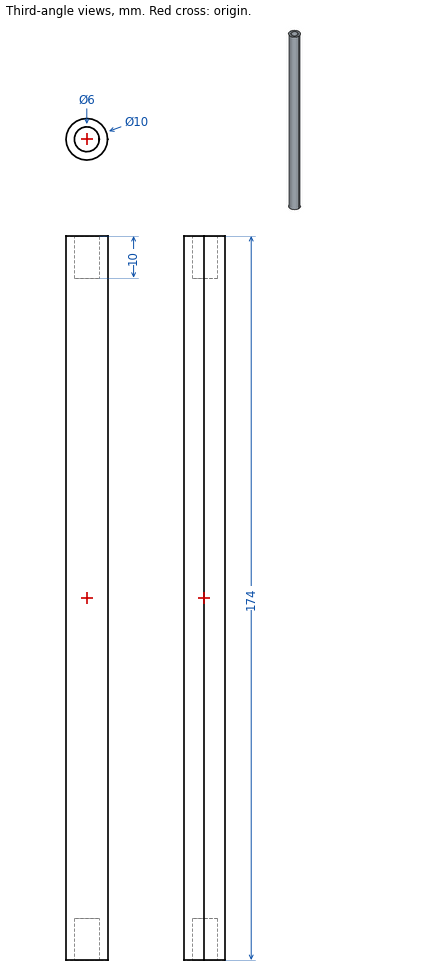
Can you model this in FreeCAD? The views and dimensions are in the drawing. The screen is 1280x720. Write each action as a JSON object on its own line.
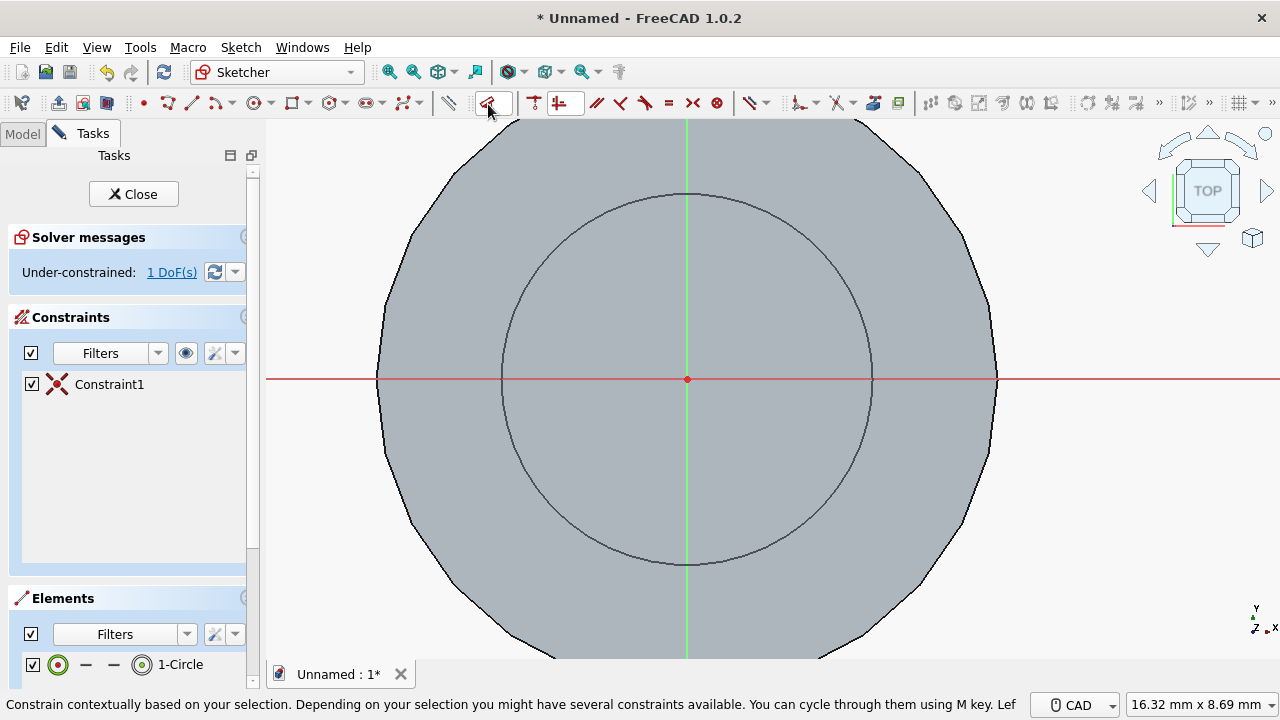
{"action": "left_click", "coordinate": [818, 248]}
{"action": "left_click", "coordinate": [841, 225]}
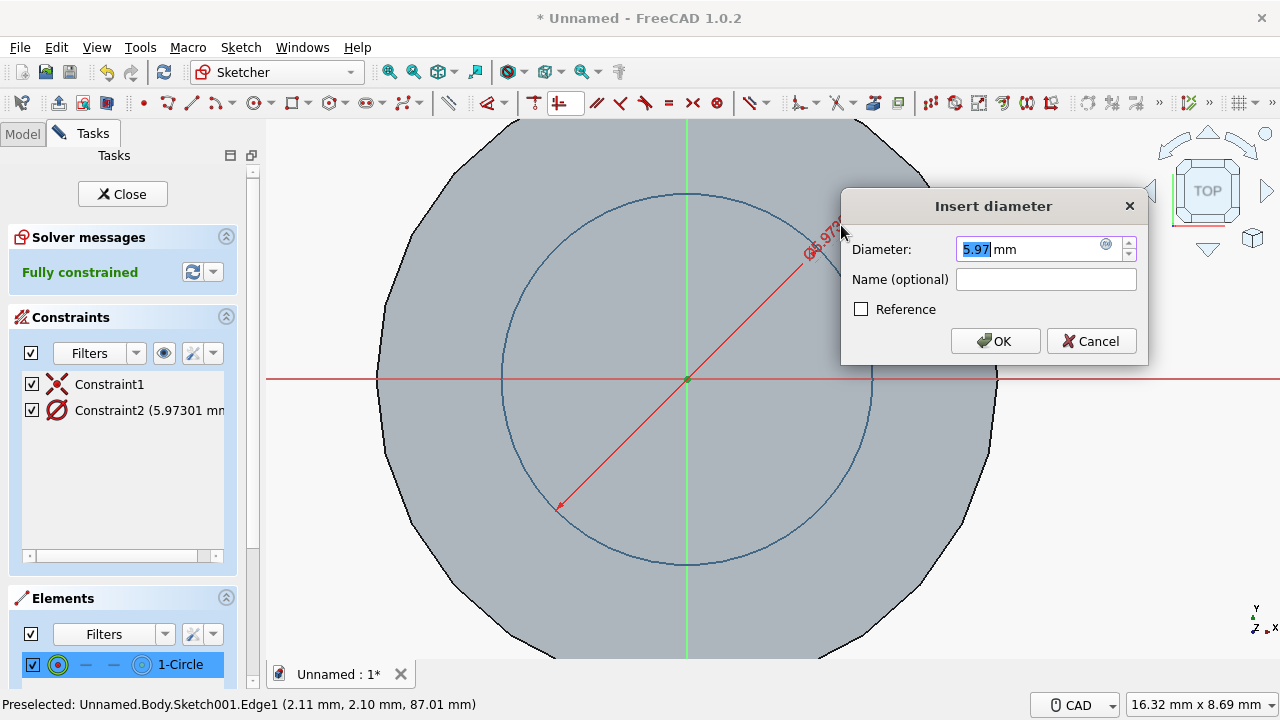
{"action": "type", "text": "6"}
{"action": "key", "text": "Return"}
{"action": "key", "text": "Escape"}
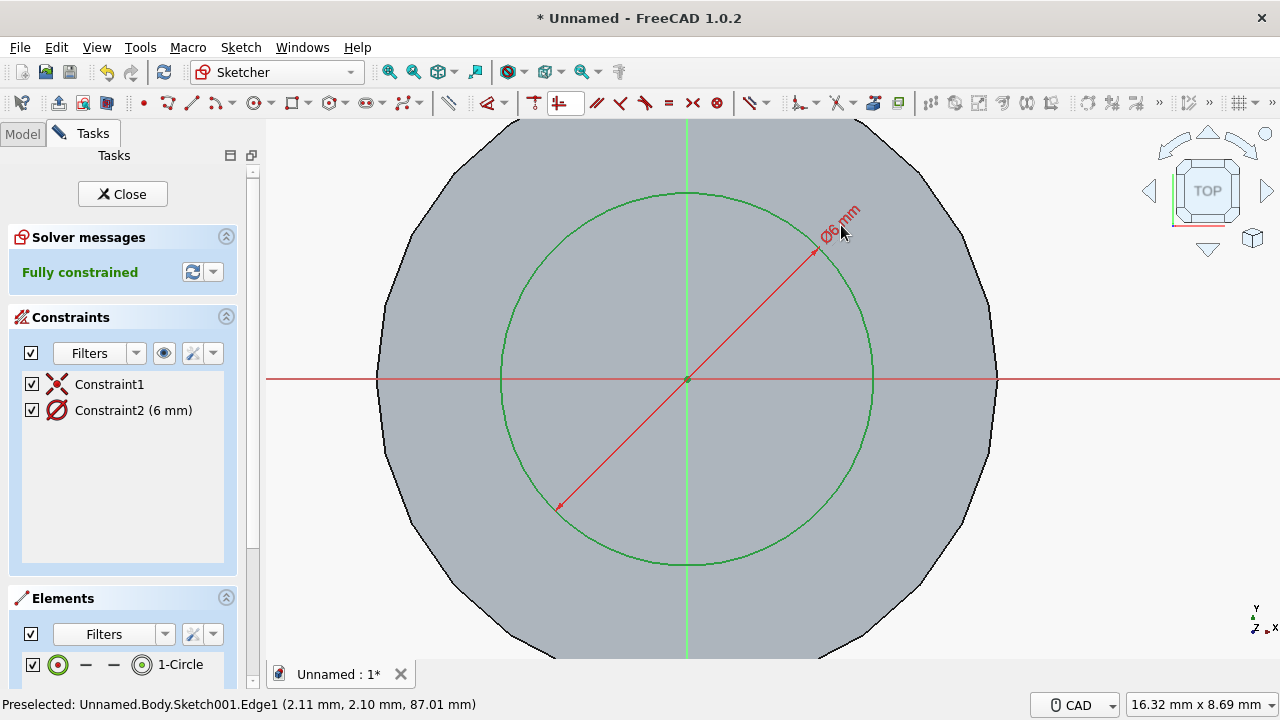
{"action": "left_click", "coordinate": [123, 194]}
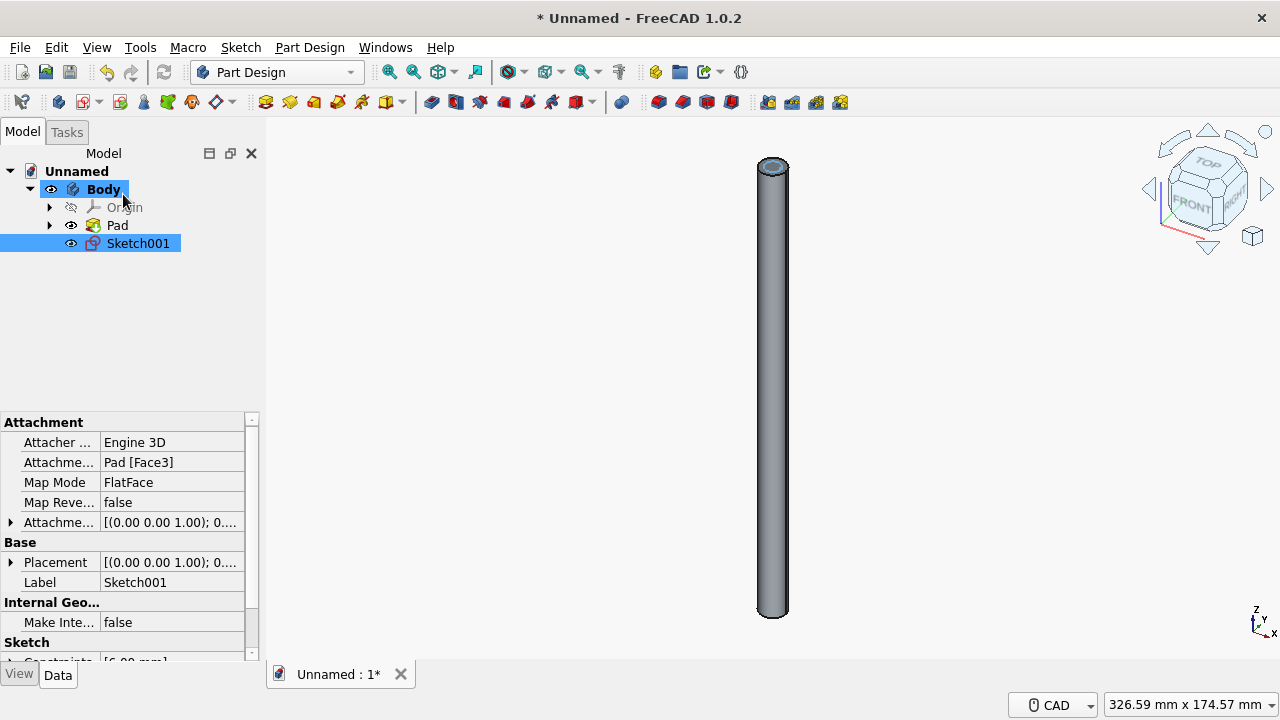
{"action": "left_click", "coordinate": [432, 102]}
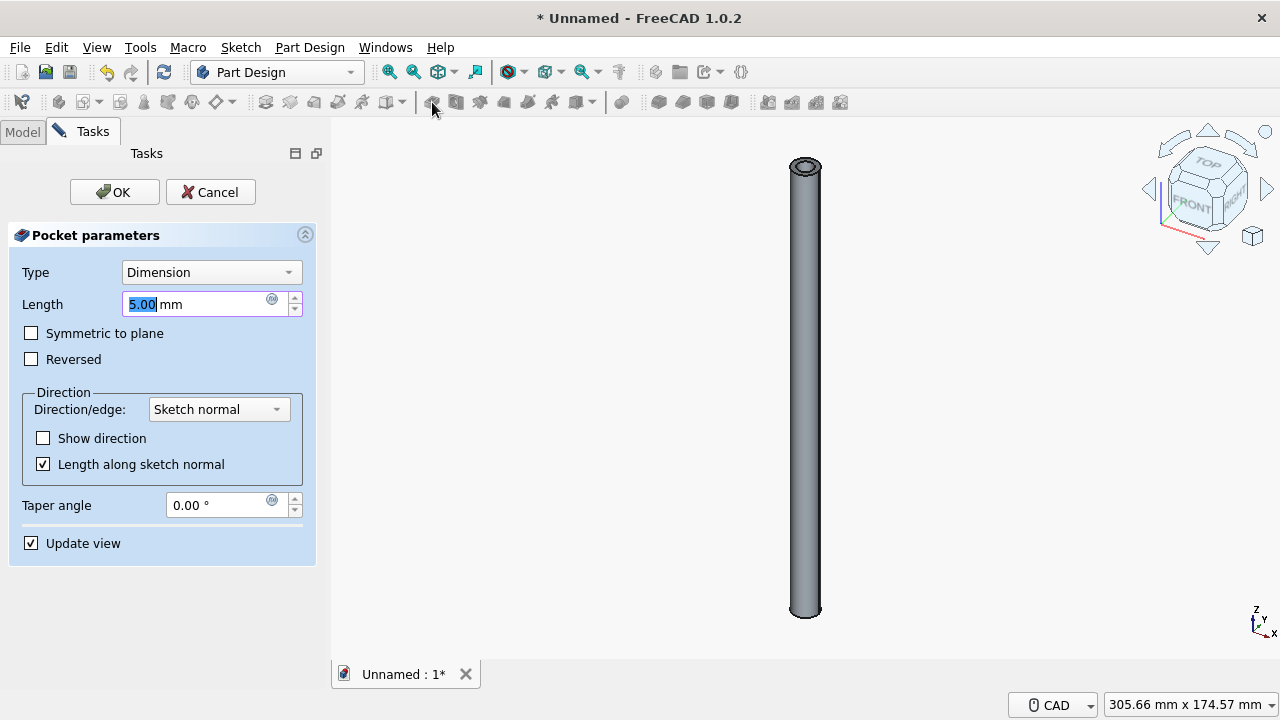
{"action": "type", "text": "10"}
{"action": "key", "text": "Tab"}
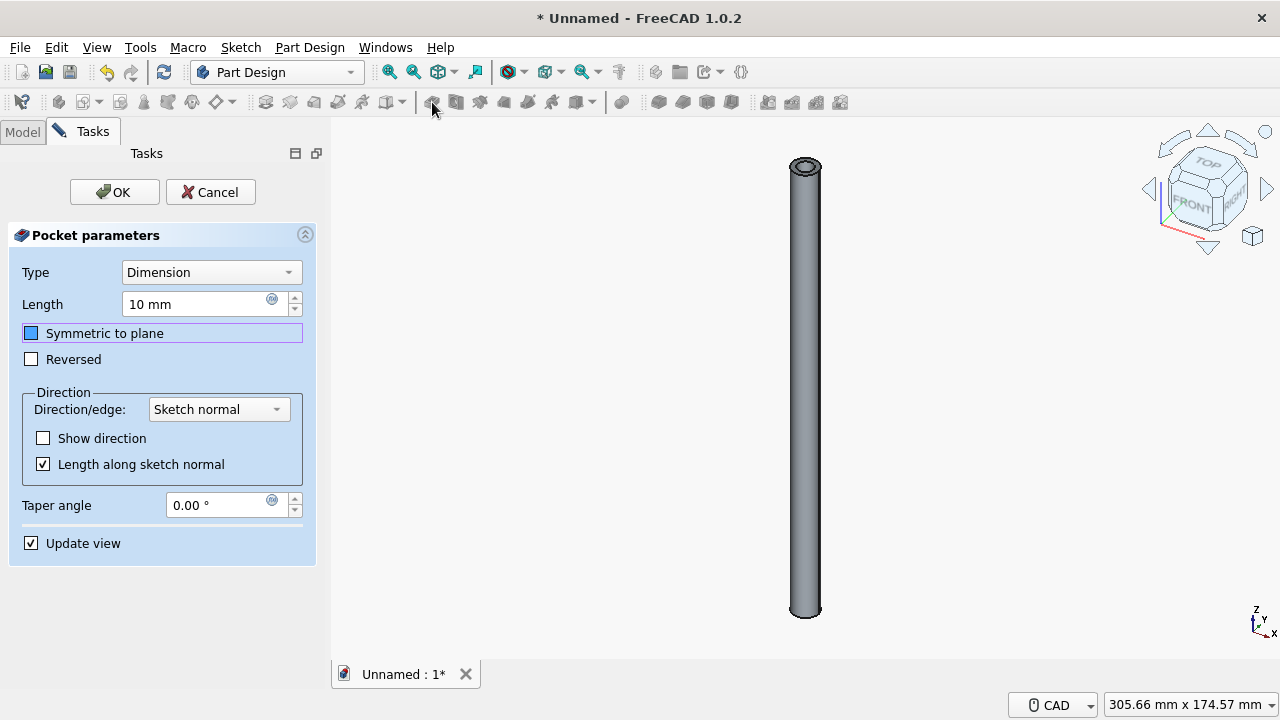
{"action": "left_click", "coordinate": [115, 192]}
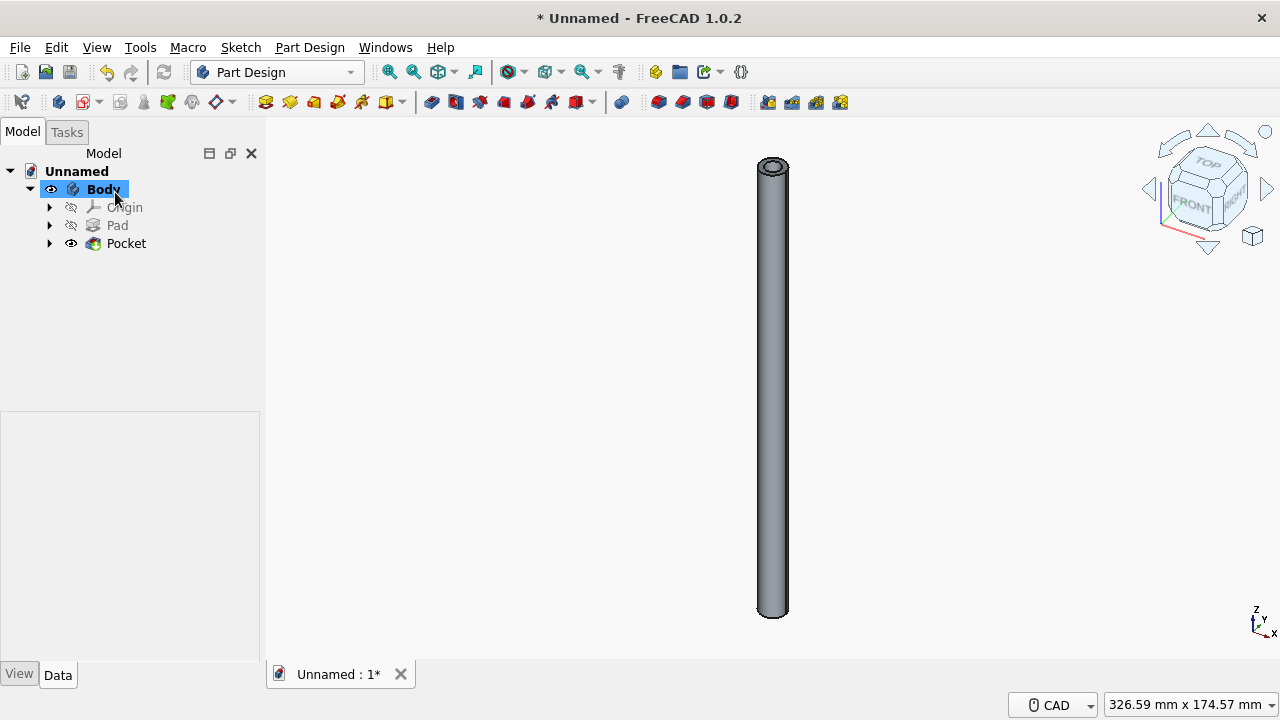
{"action": "left_click", "coordinate": [116, 243]}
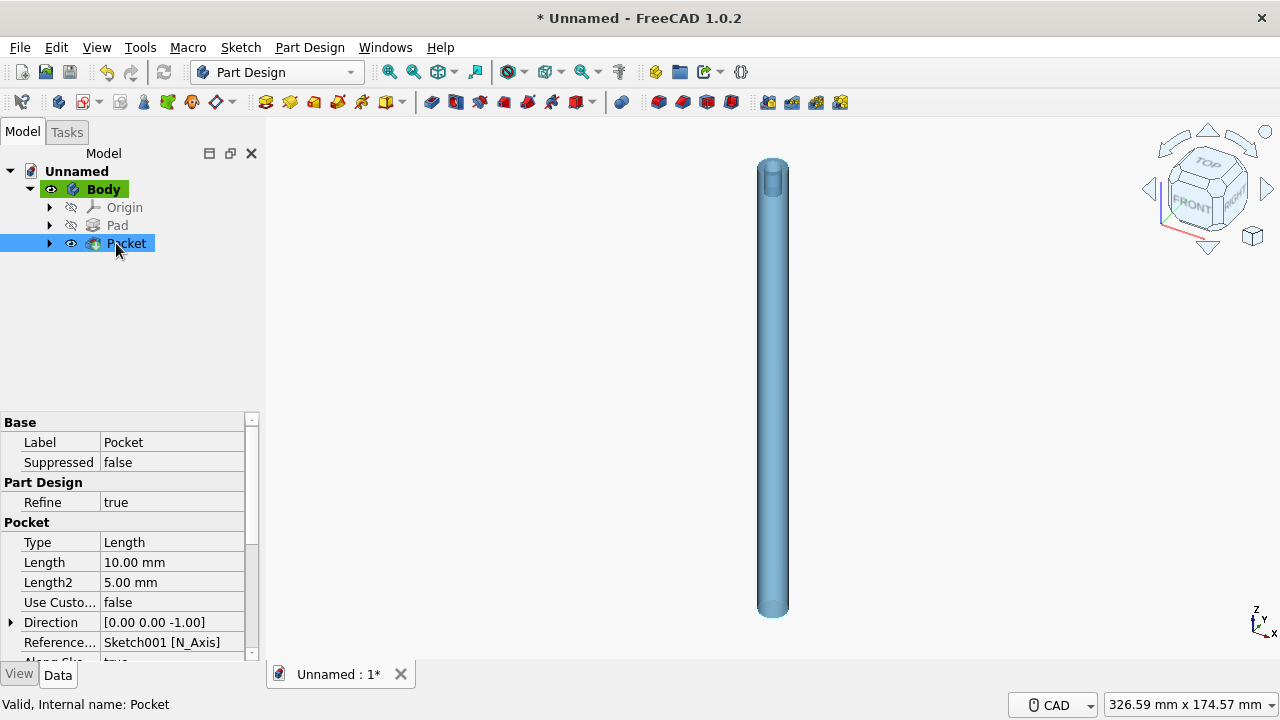
{"action": "left_click", "coordinate": [768, 102]}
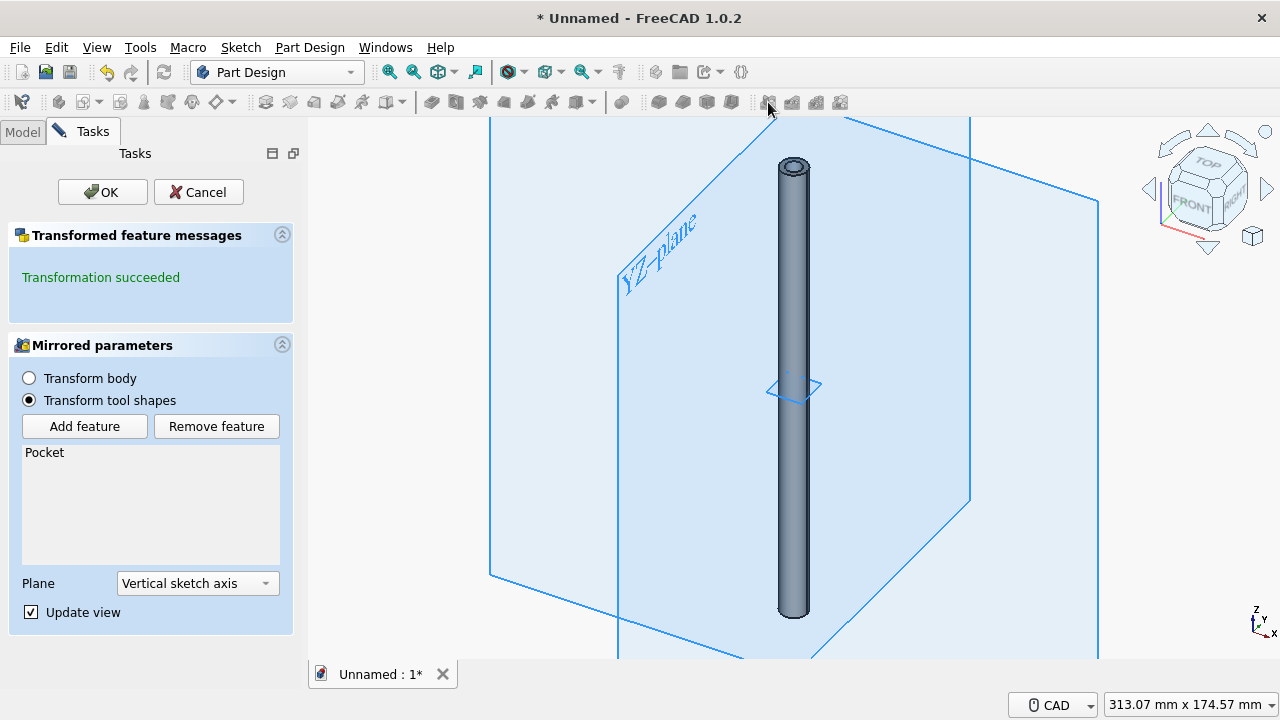
{"action": "left_click", "coordinate": [198, 584]}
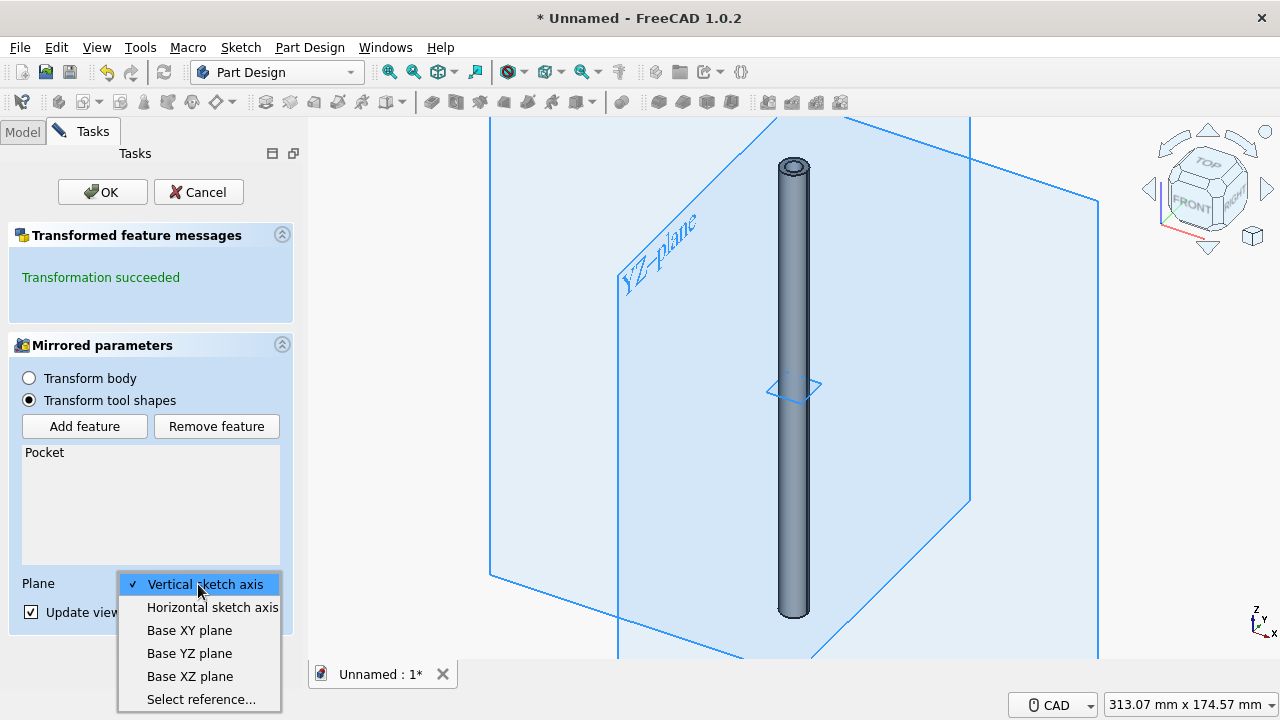
{"action": "left_click", "coordinate": [198, 630]}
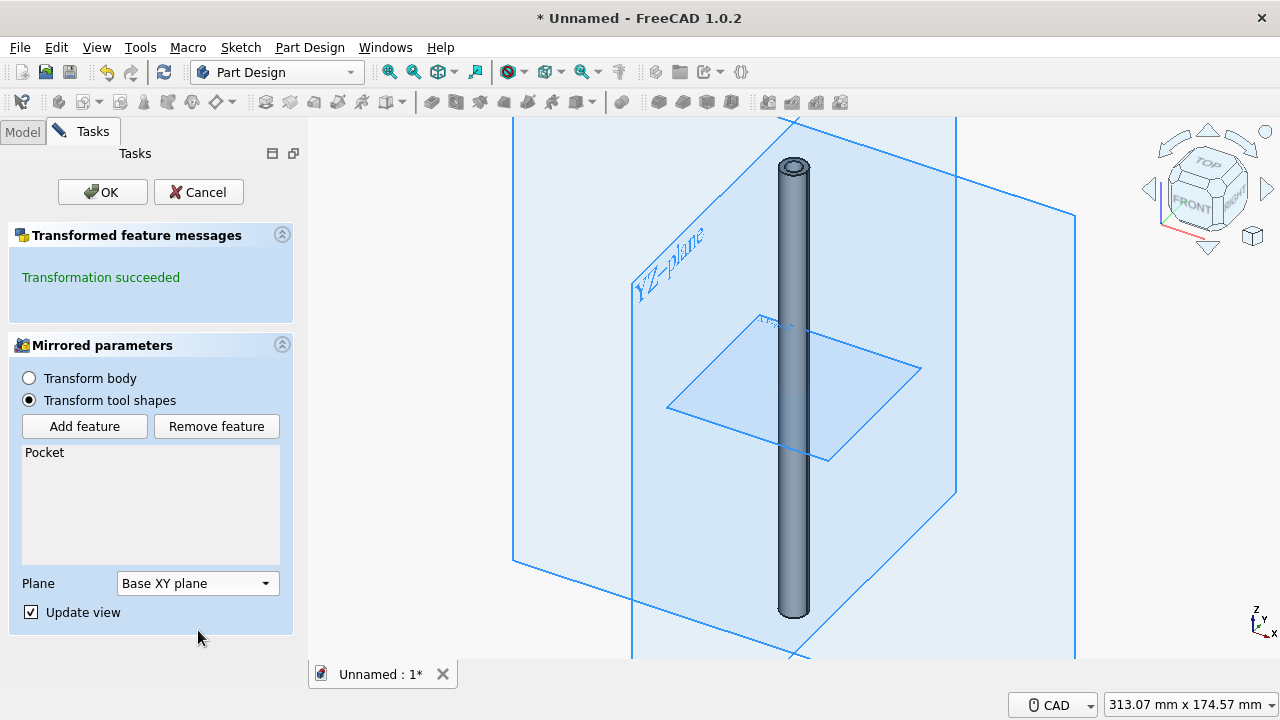
{"action": "left_click", "coordinate": [103, 192]}